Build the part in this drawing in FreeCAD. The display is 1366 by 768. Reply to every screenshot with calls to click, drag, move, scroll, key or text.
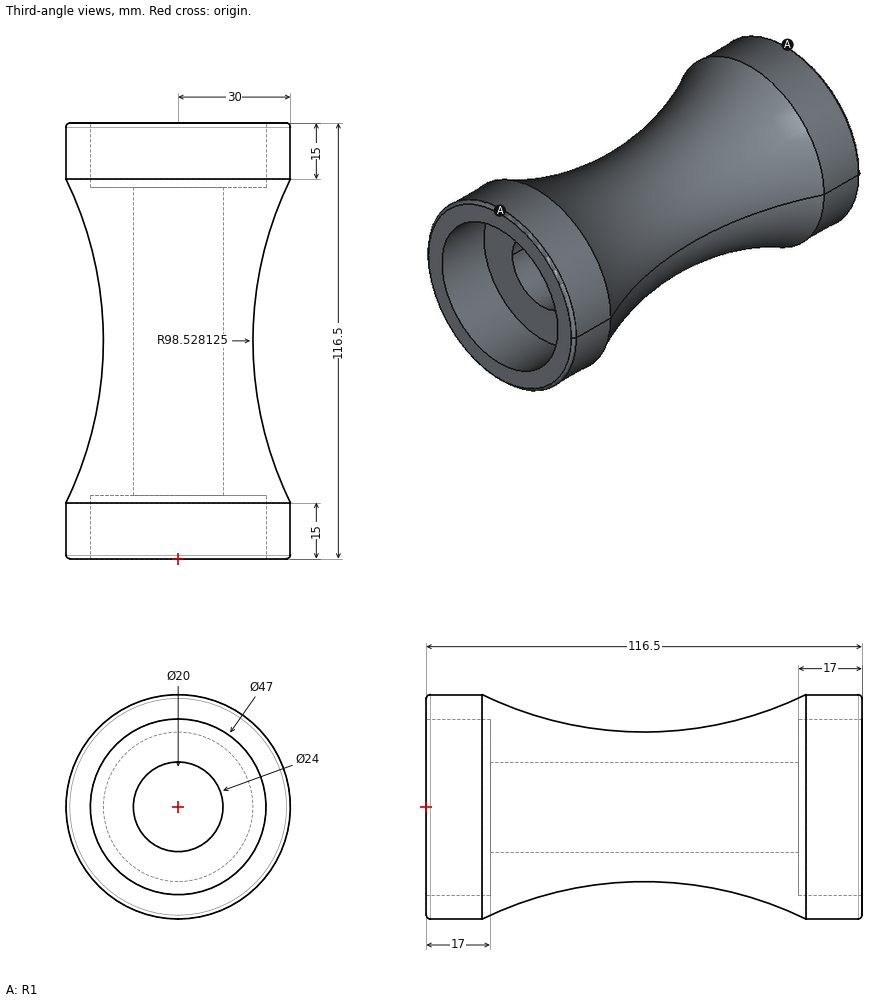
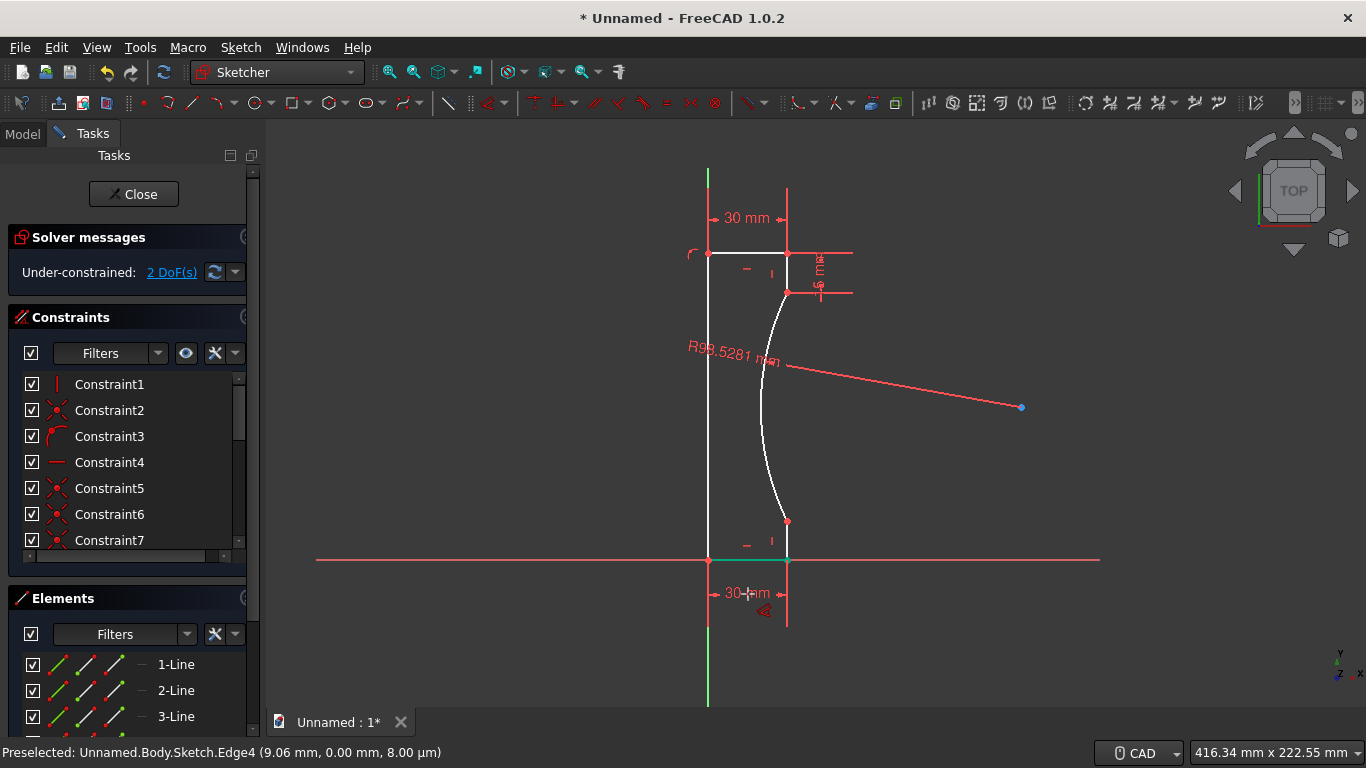
click(787, 549)
click(821, 541)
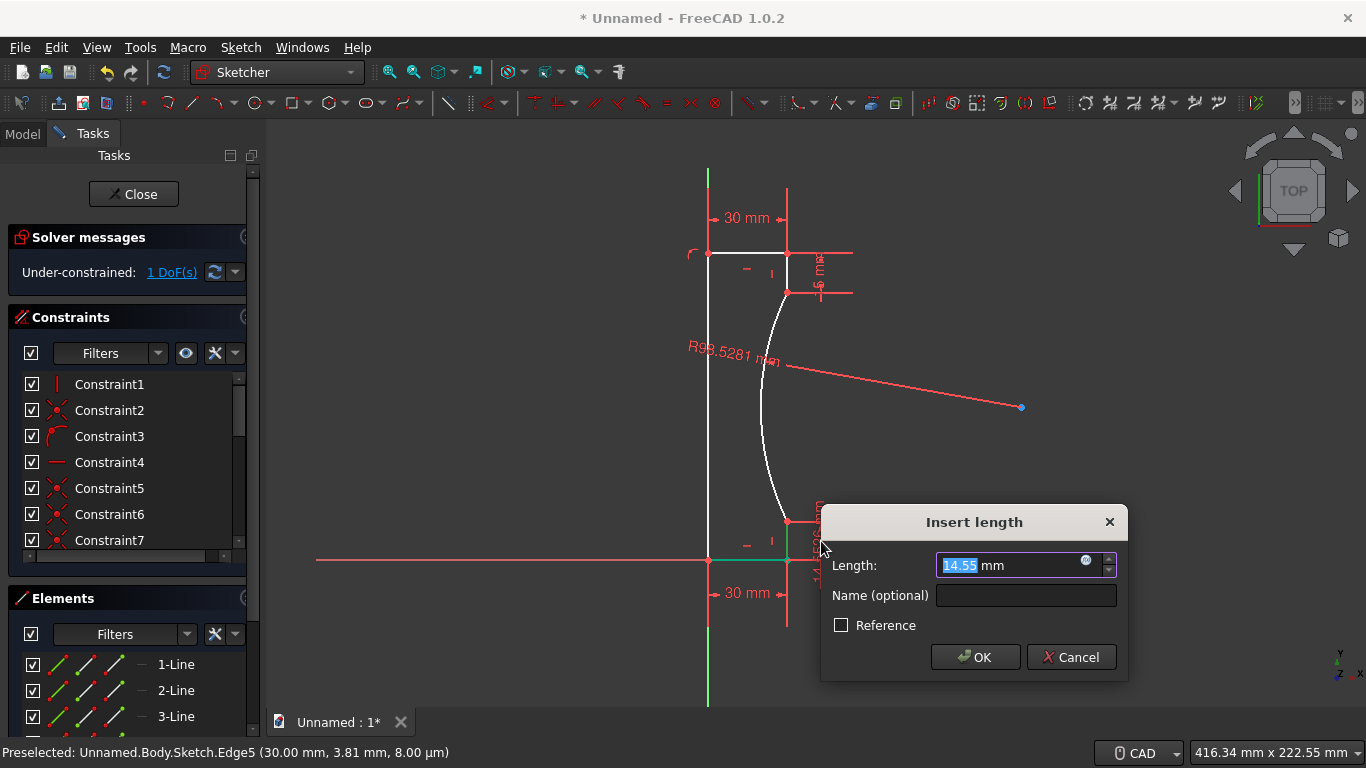
text(15)
key(Return)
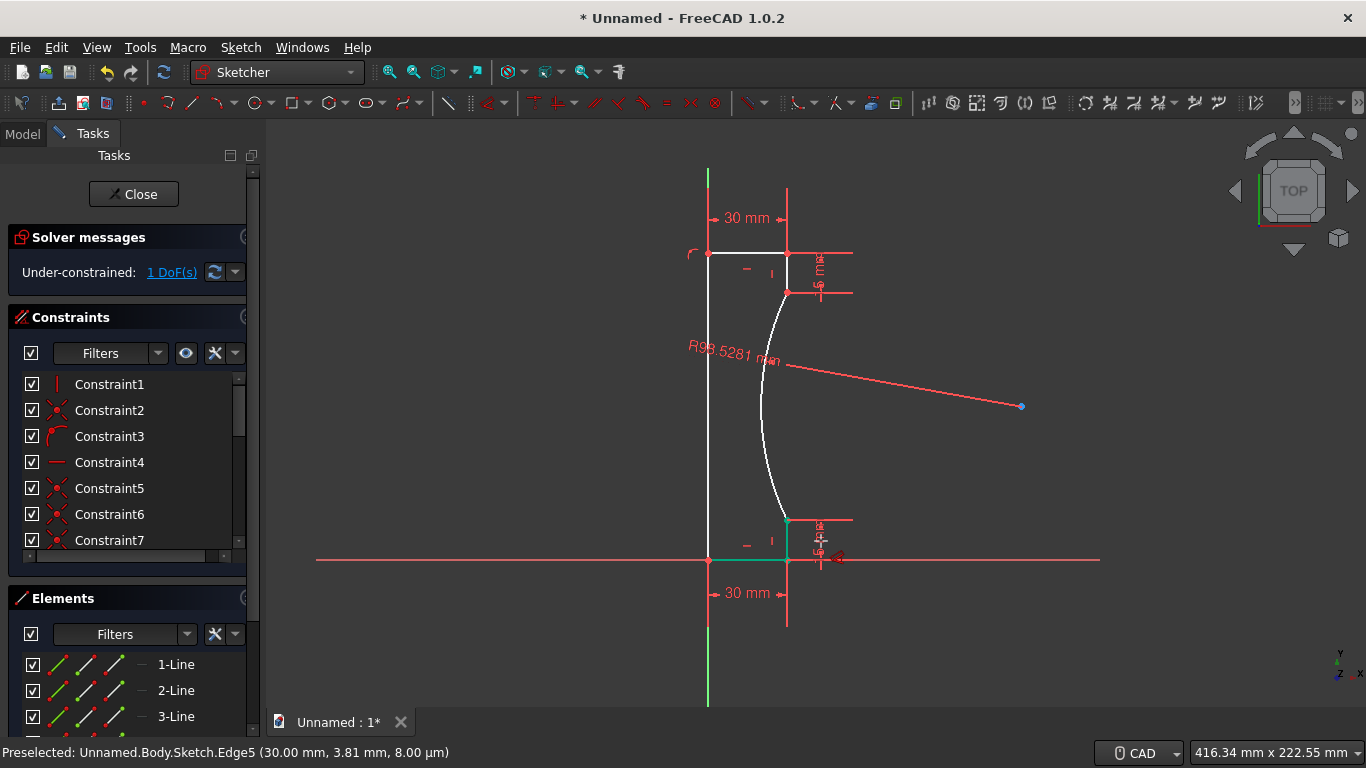
click(708, 345)
click(674, 407)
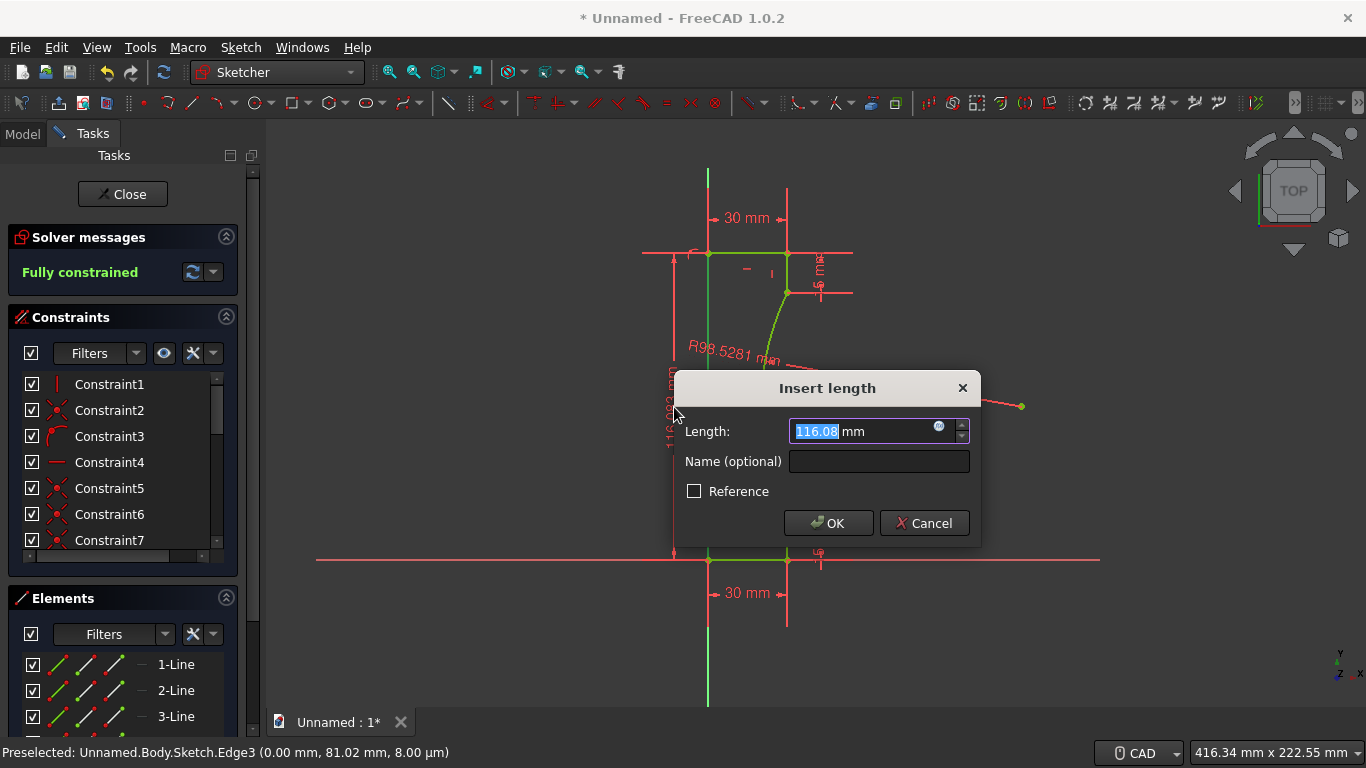
text(116.5)
key(Return)
key(Escape)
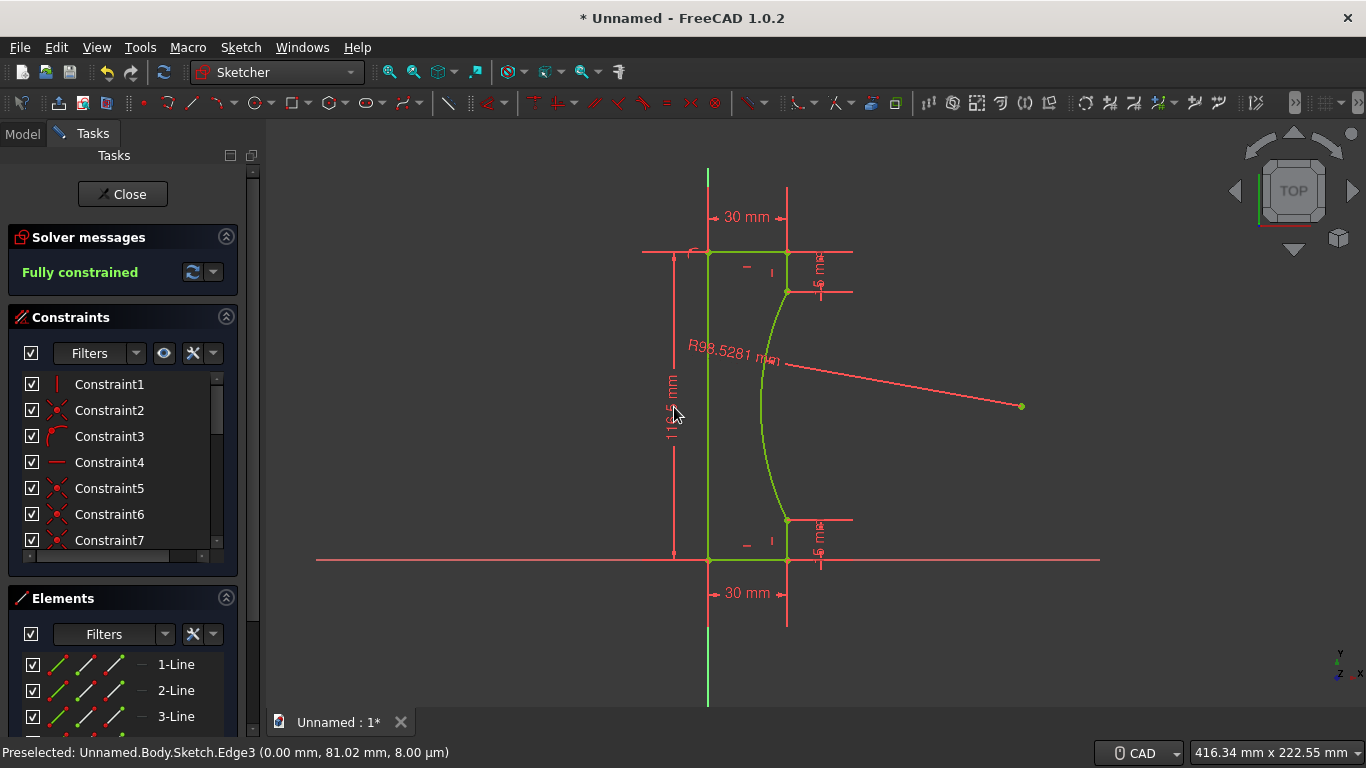
click(123, 194)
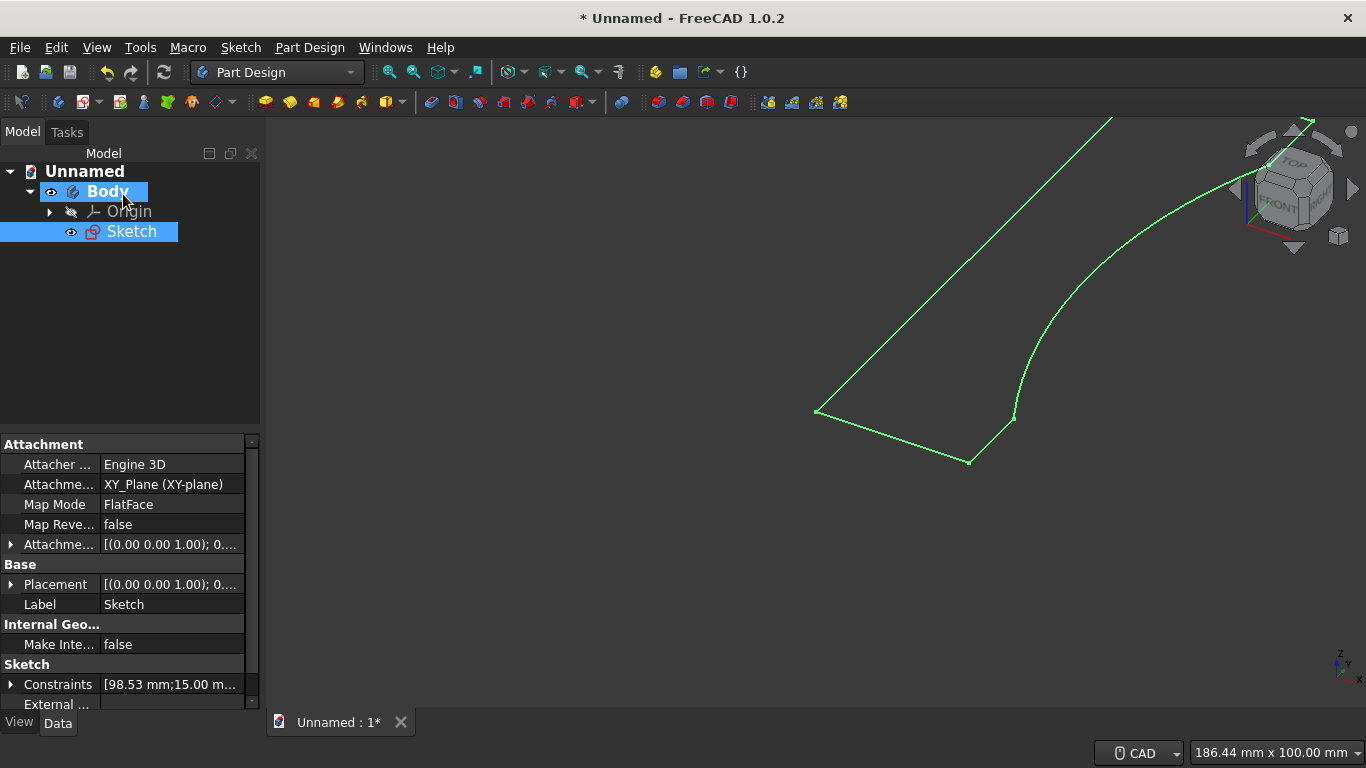
click(290, 102)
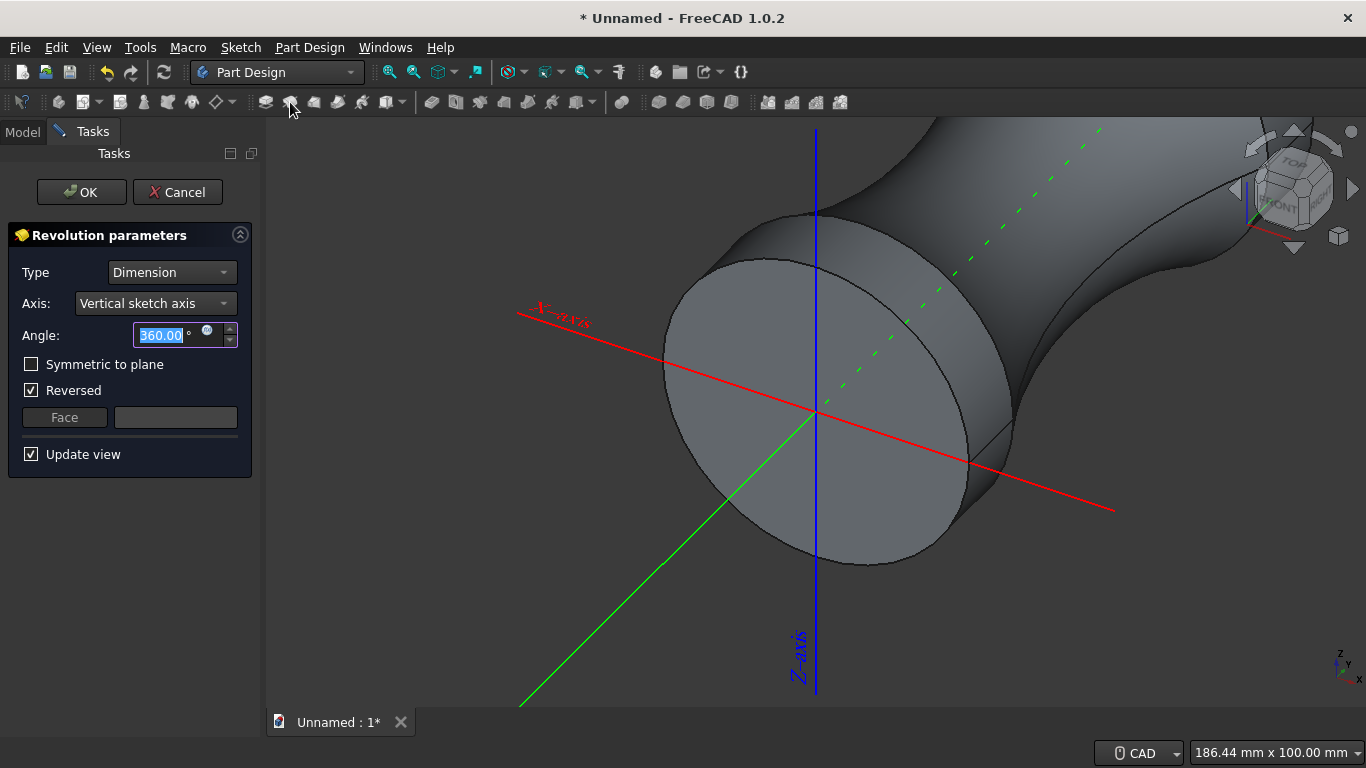
click(82, 192)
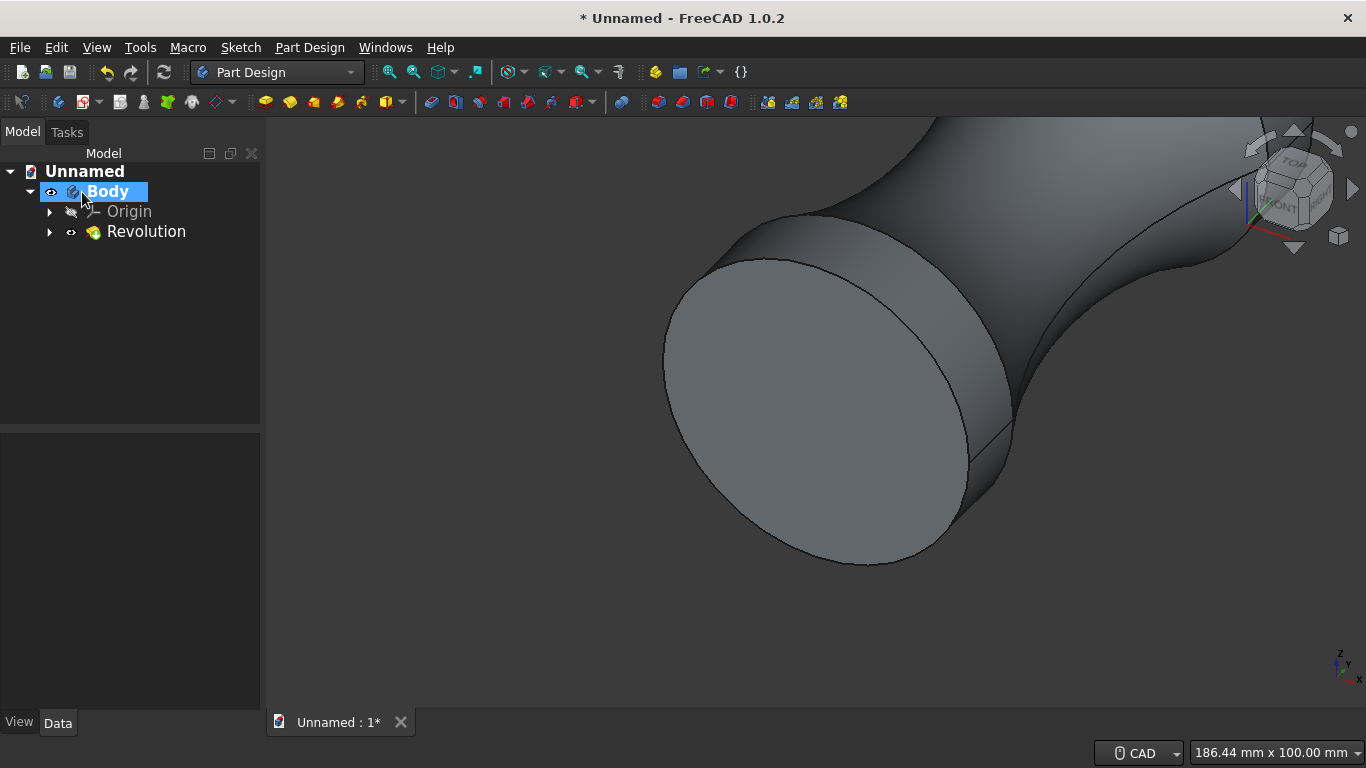
click(390, 72)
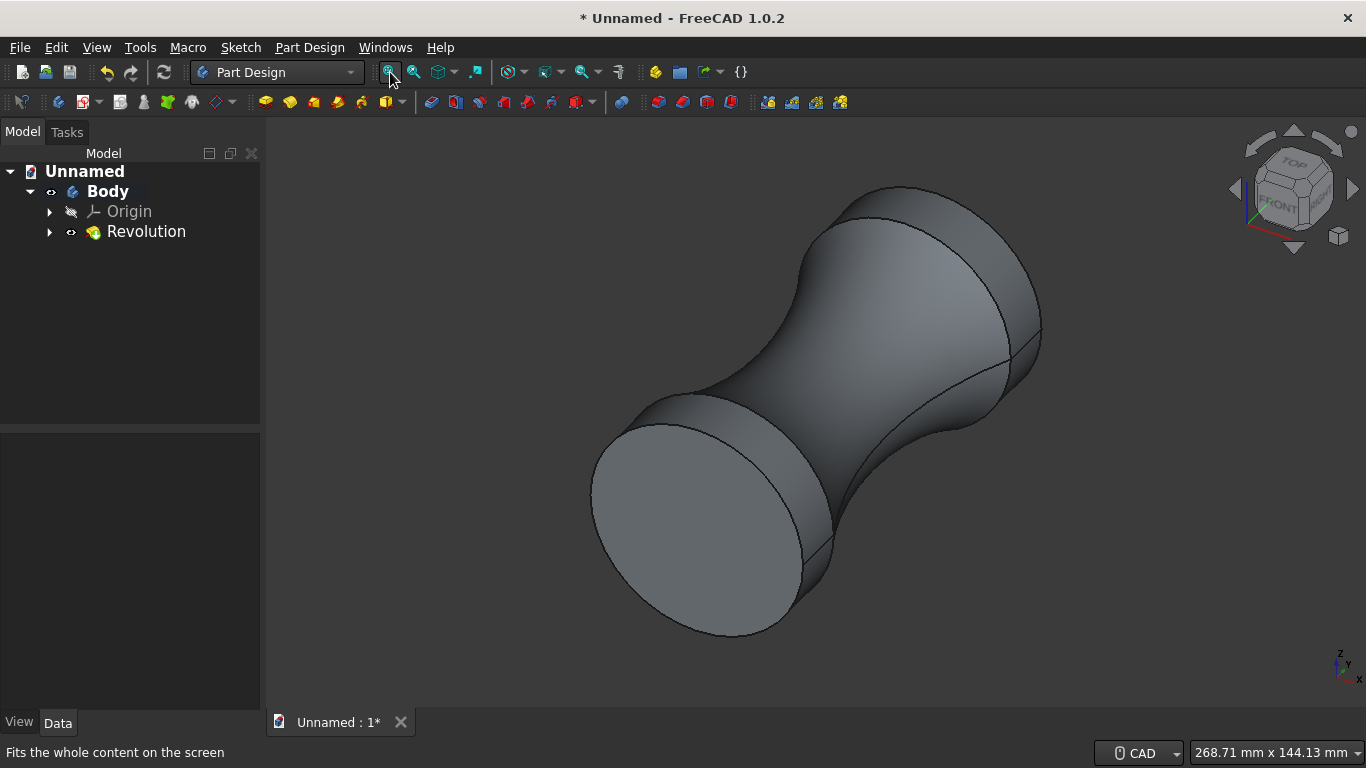
key(4)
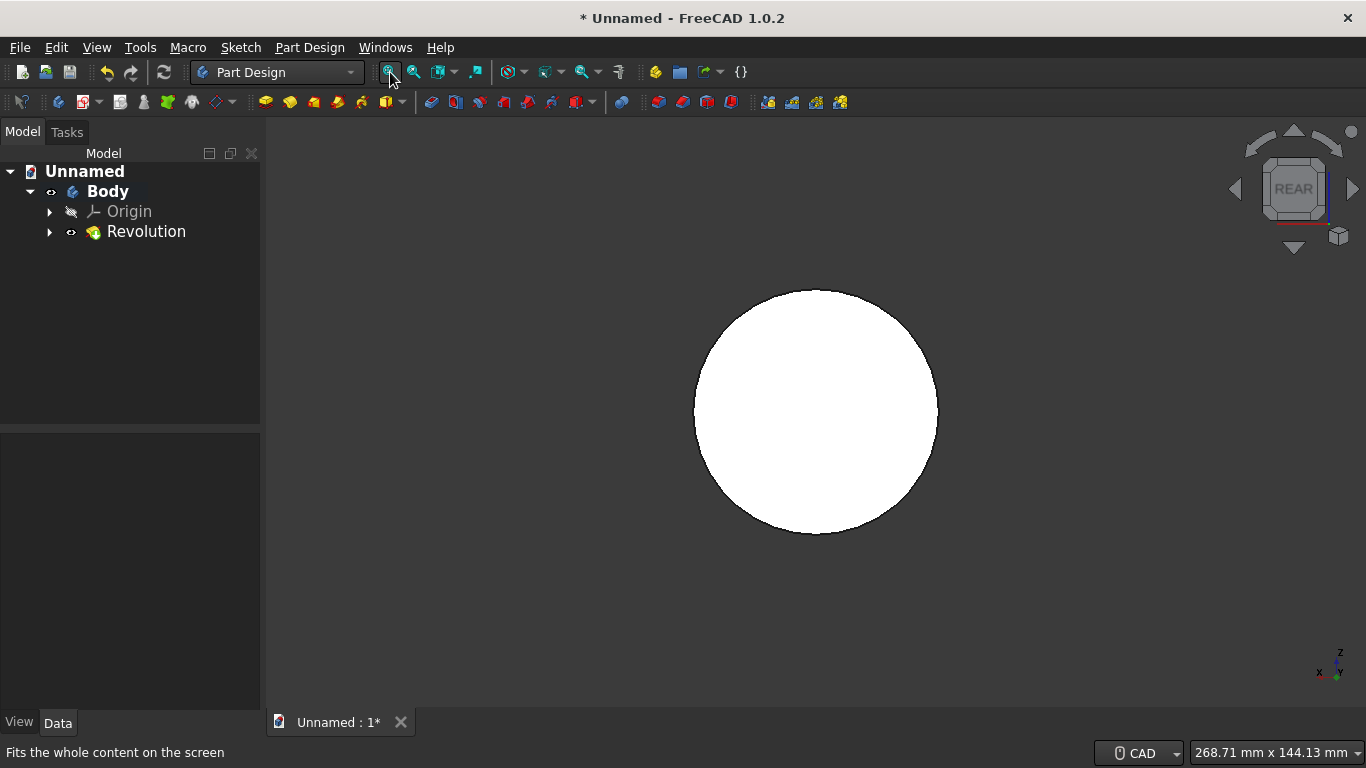
click(390, 72)